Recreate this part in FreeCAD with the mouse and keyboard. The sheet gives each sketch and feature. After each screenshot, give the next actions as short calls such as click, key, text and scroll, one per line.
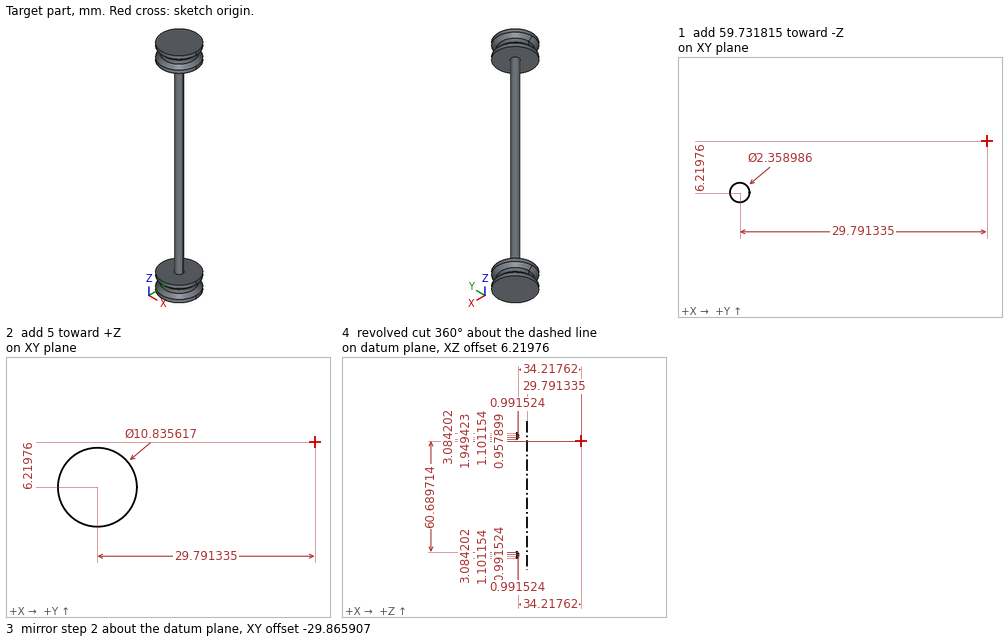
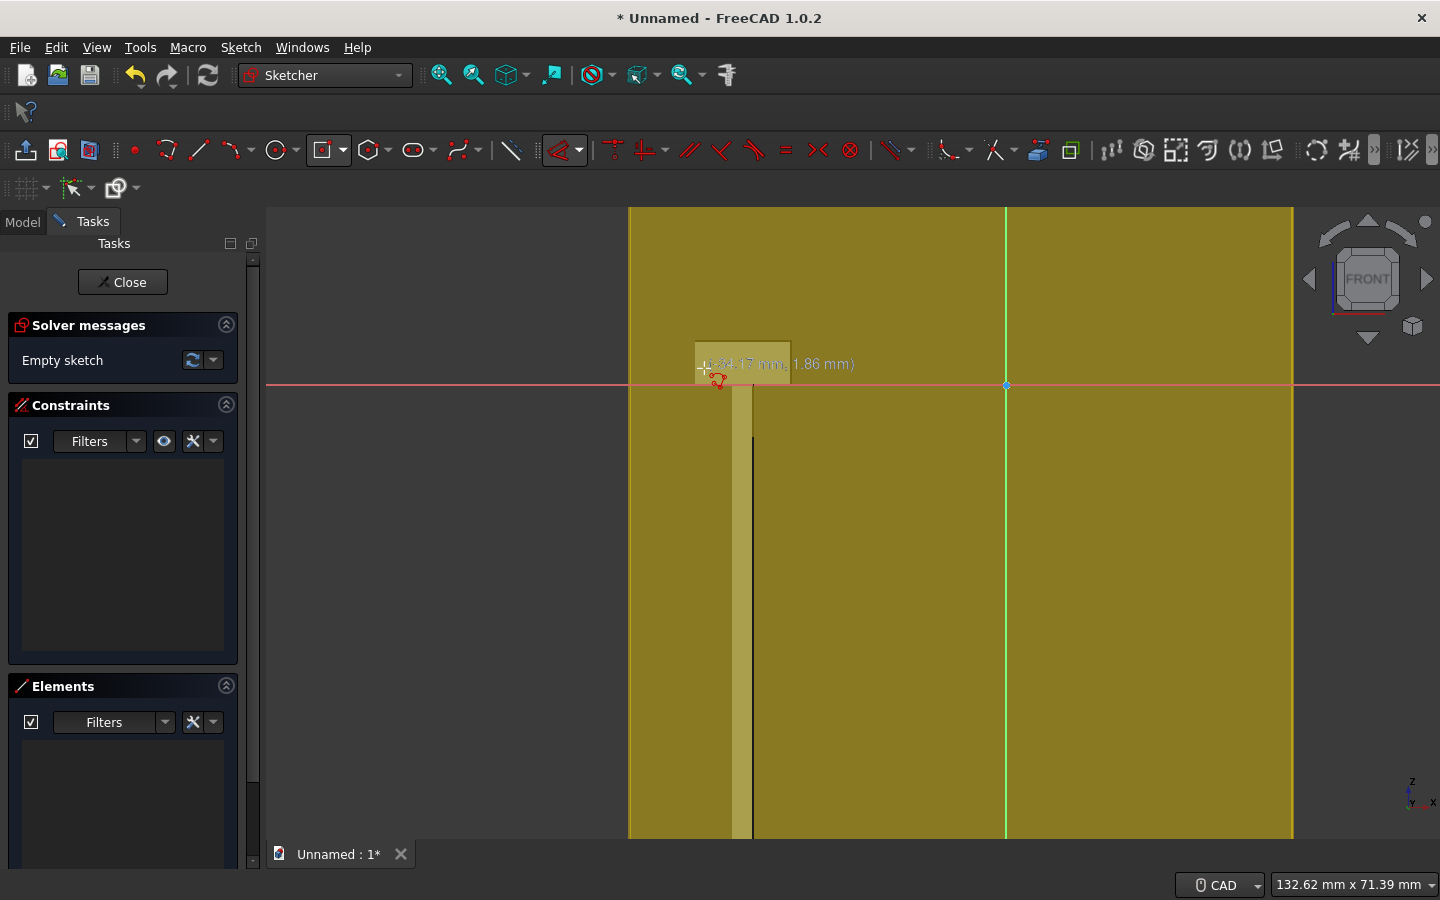
scroll(695, 377, up, 4)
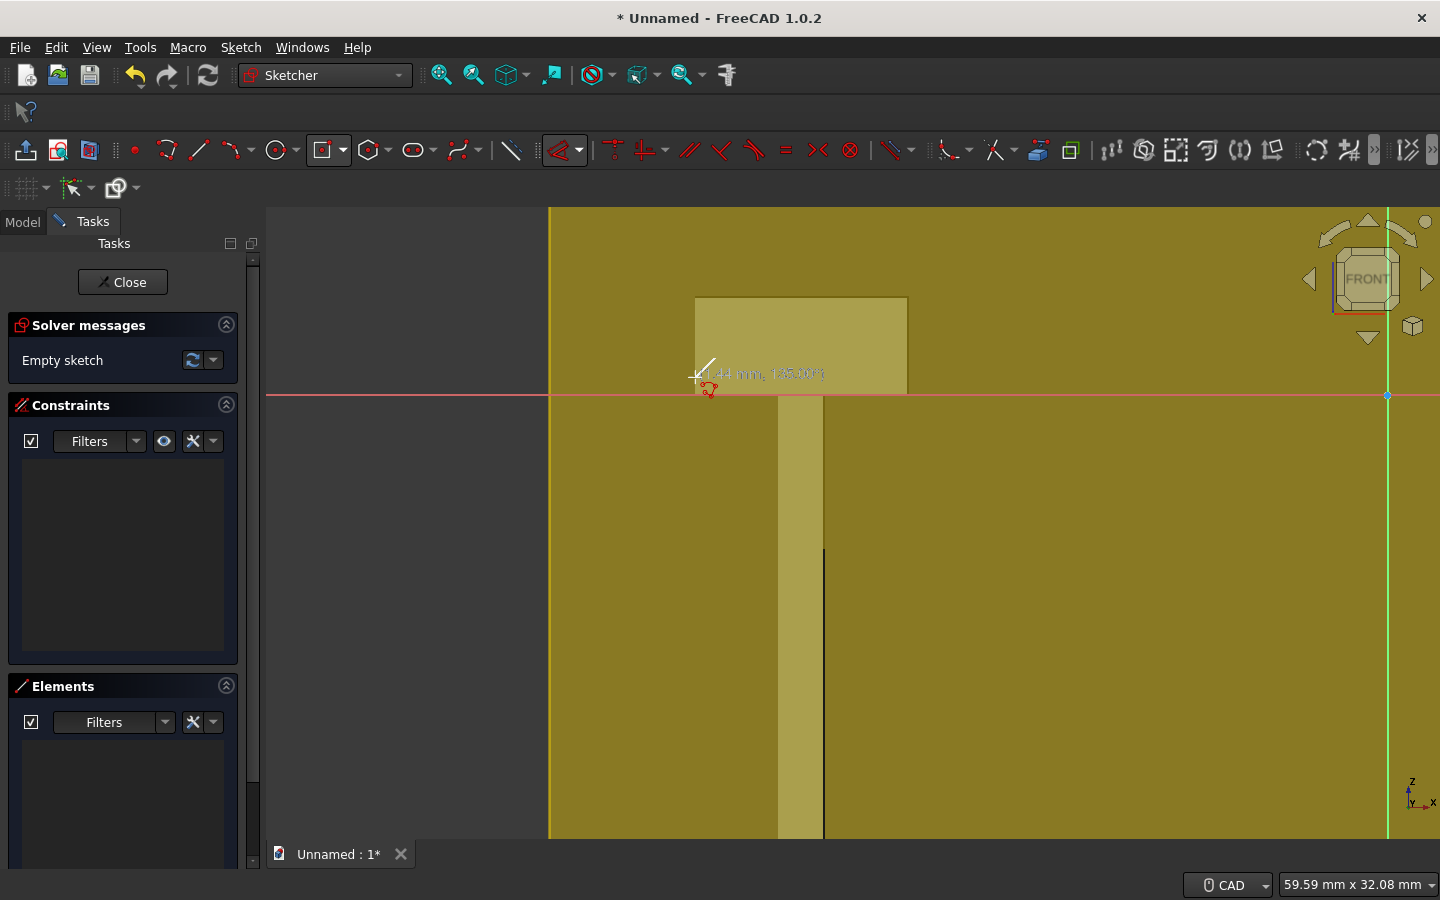
click(694, 377)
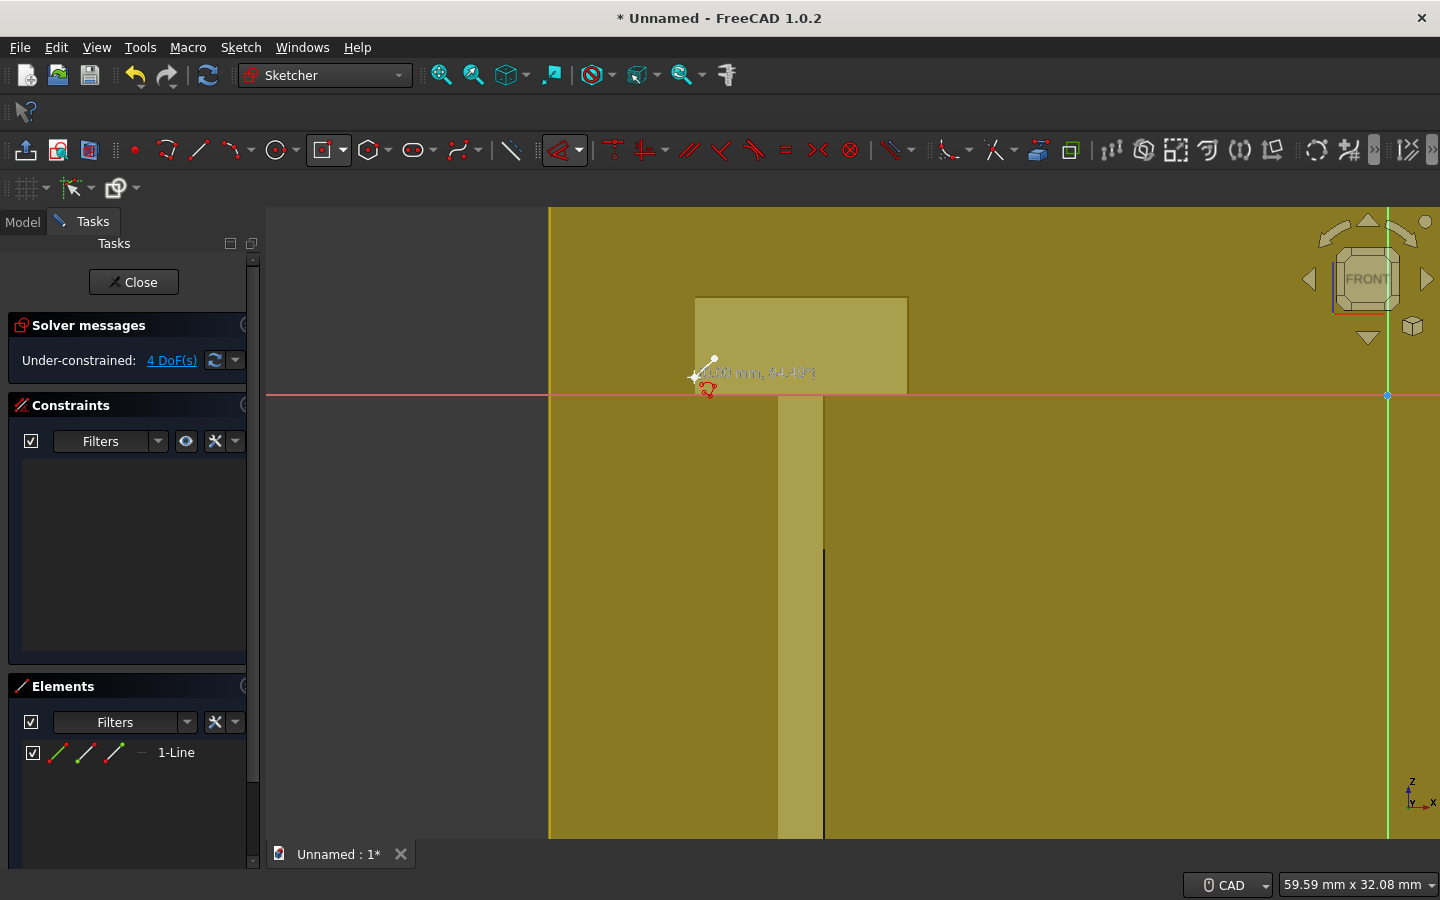
scroll(701, 372, down, 7)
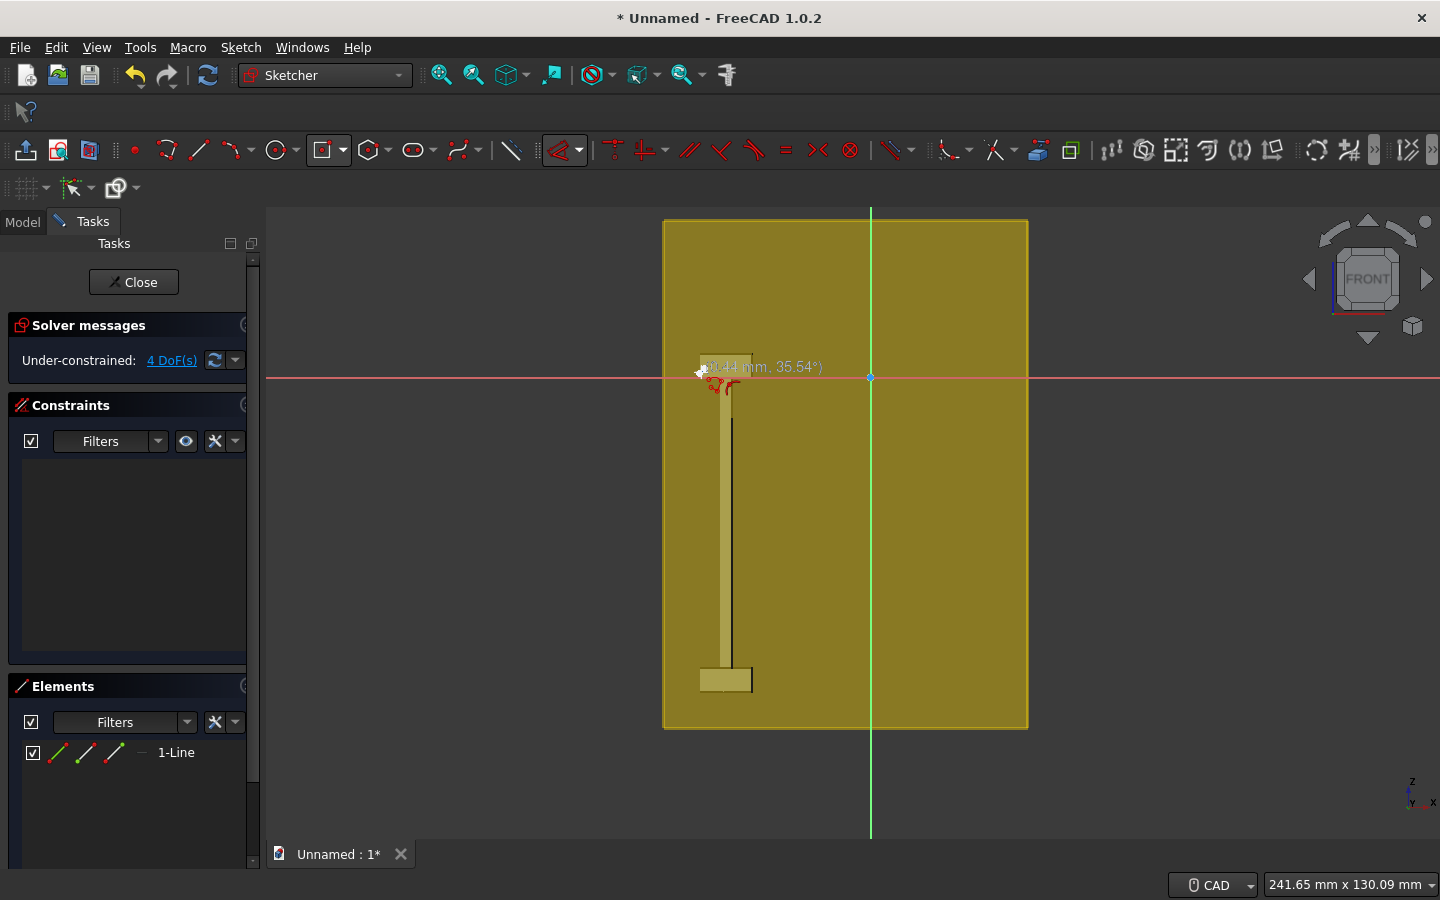
scroll(700, 358, up, 2)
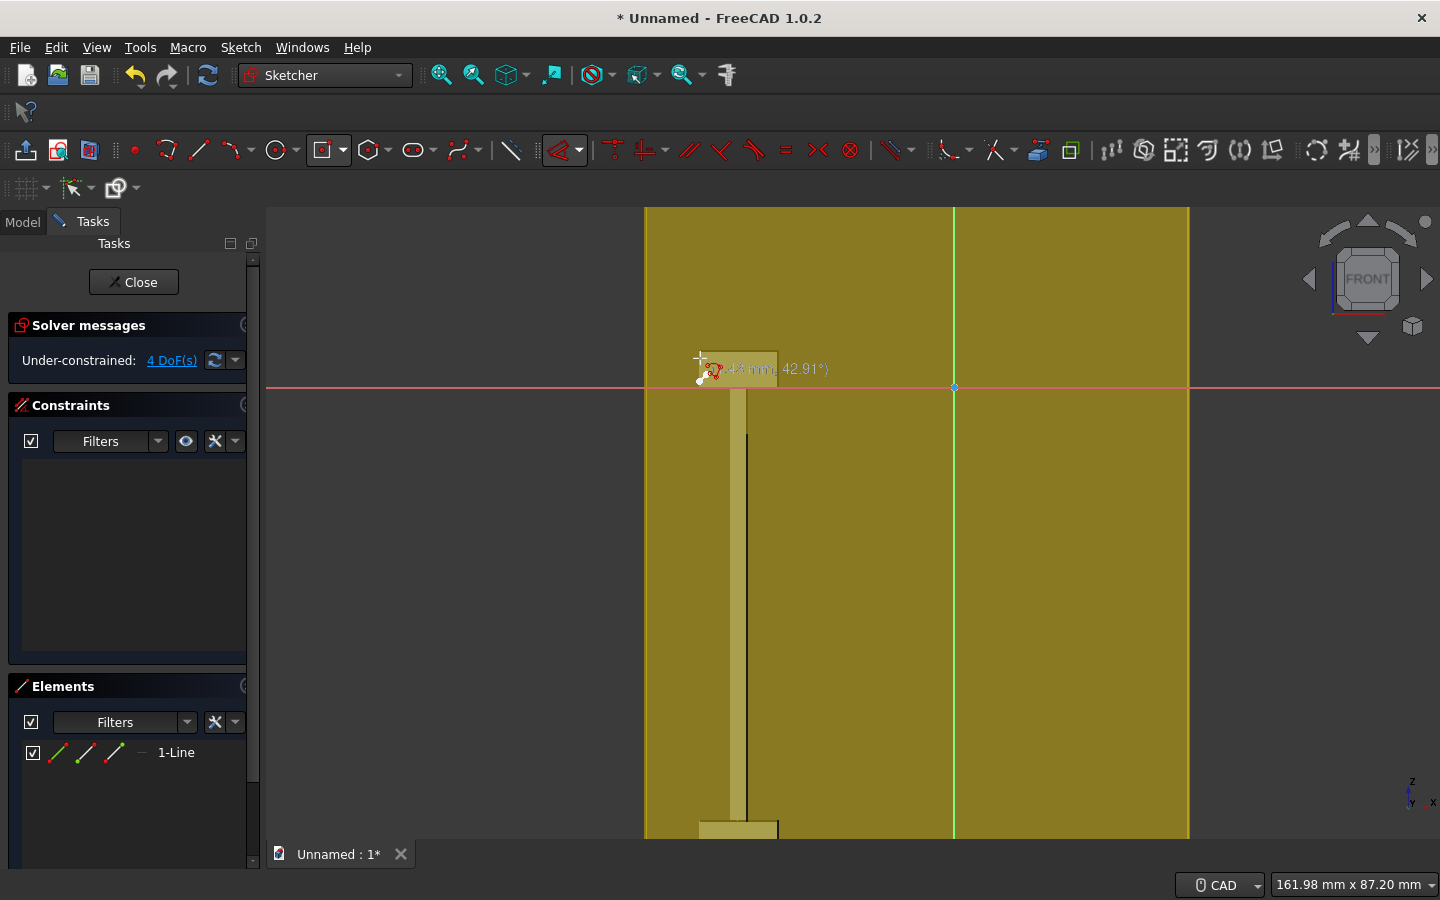
click(699, 358)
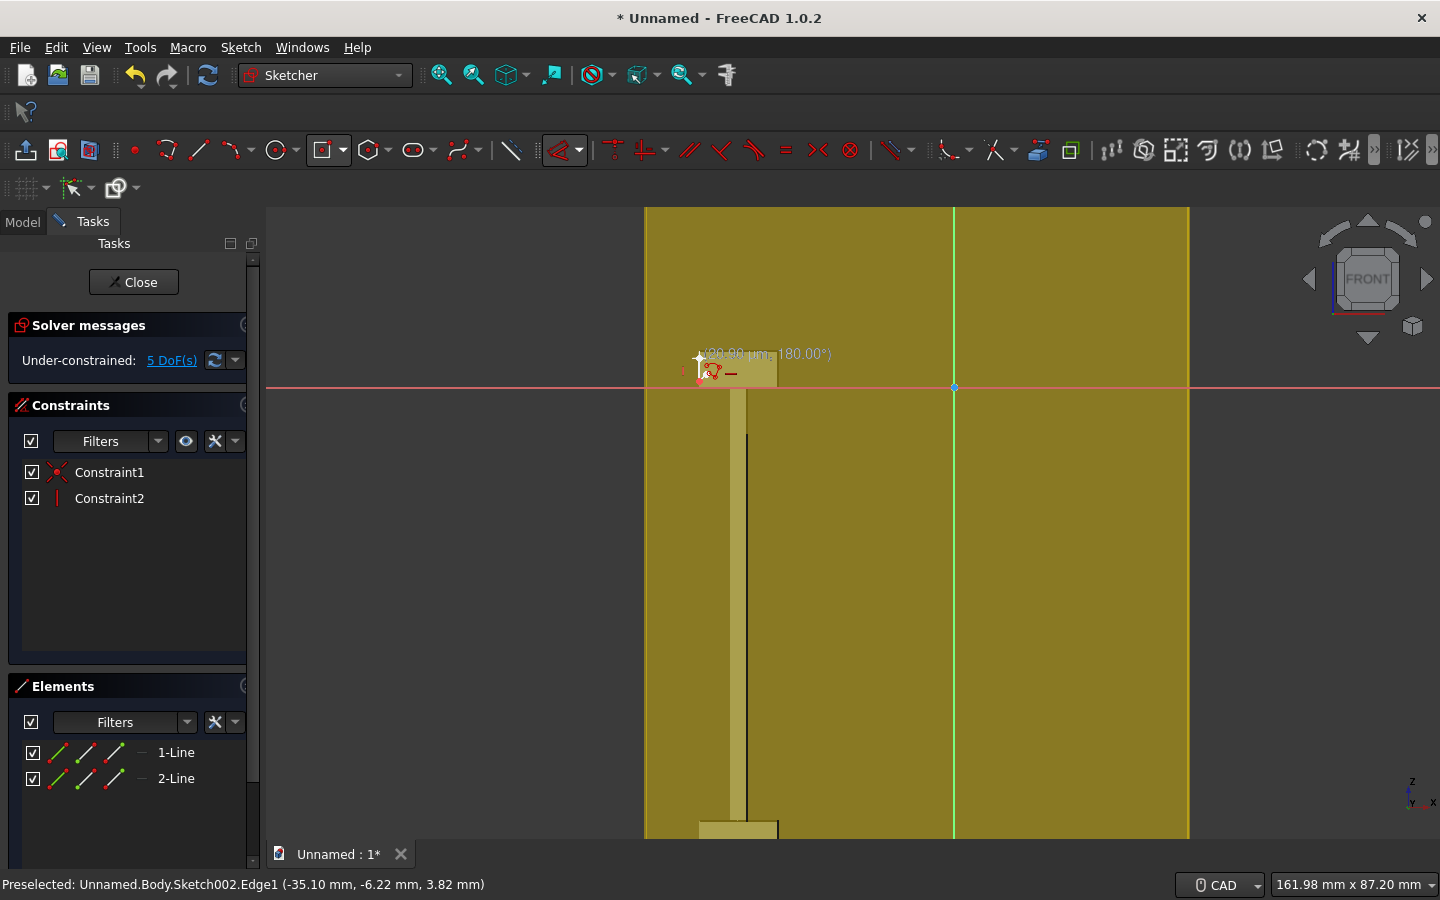
scroll(706, 366, up, 4)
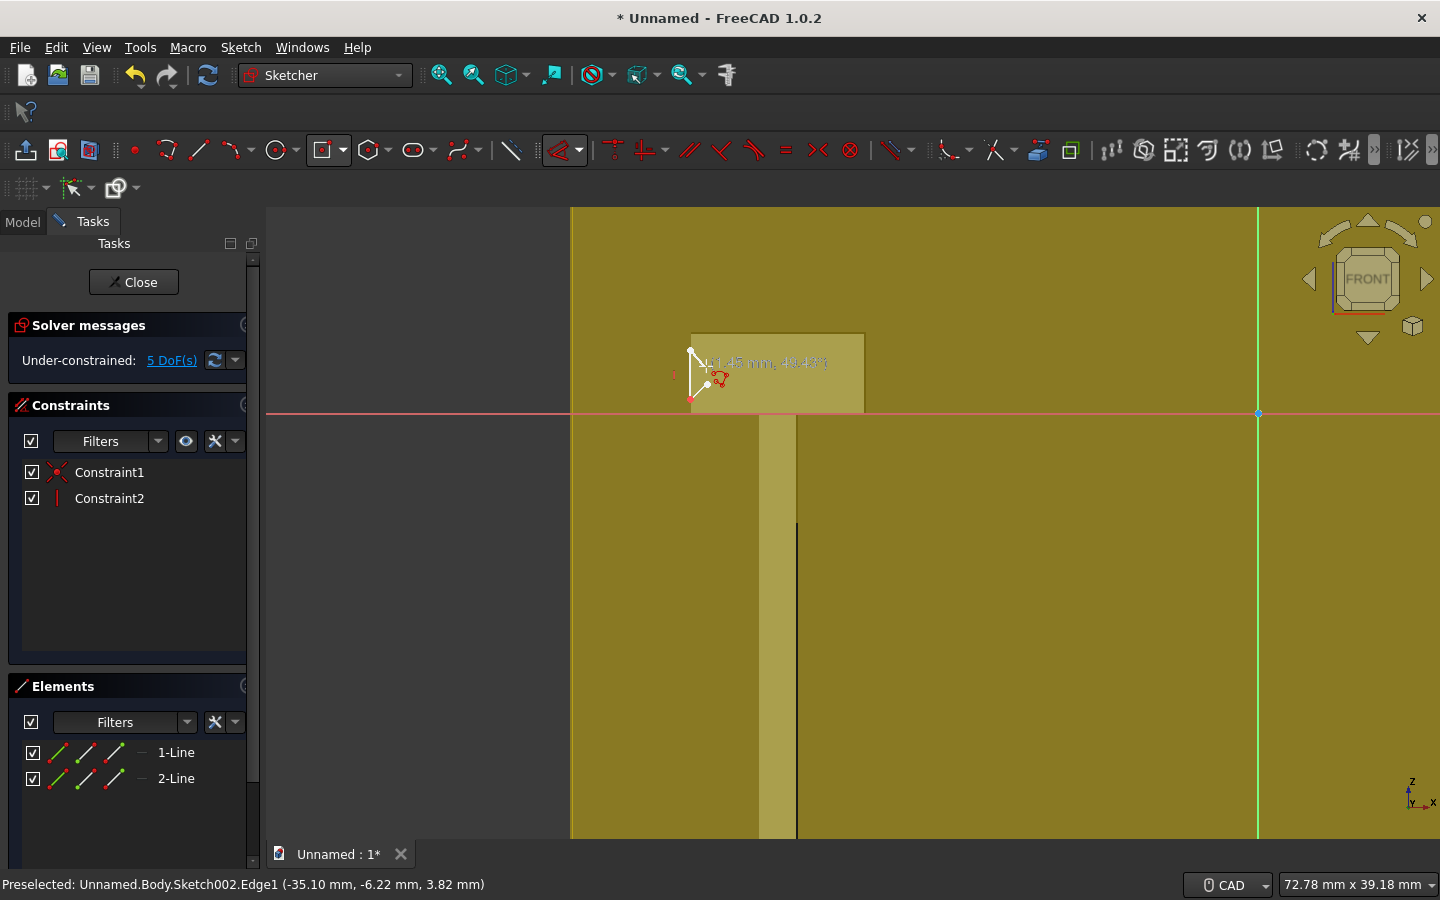
click(706, 365)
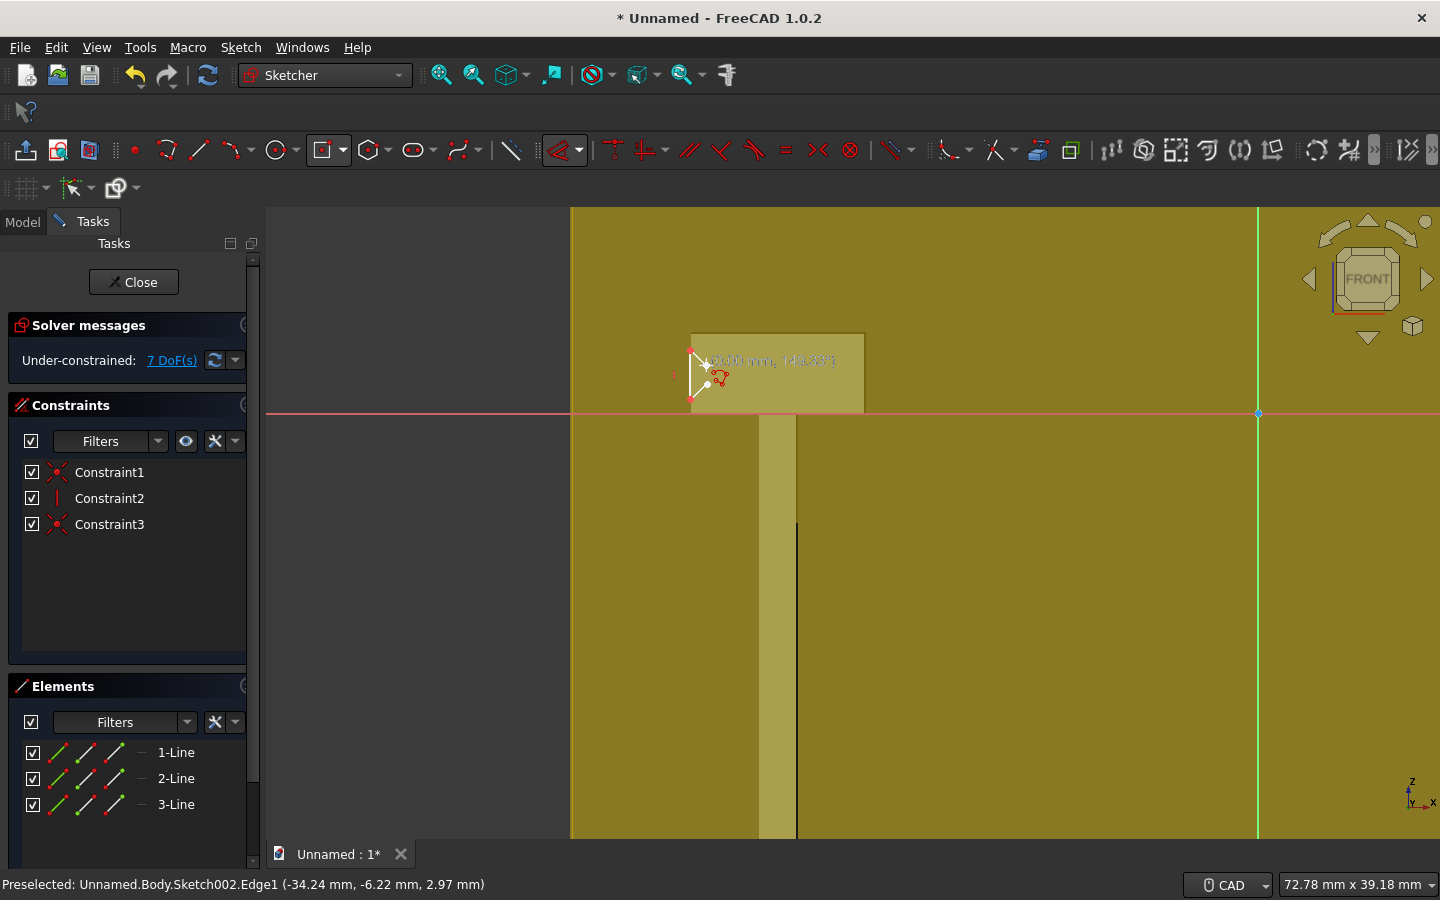
scroll(706, 382, up, 2)